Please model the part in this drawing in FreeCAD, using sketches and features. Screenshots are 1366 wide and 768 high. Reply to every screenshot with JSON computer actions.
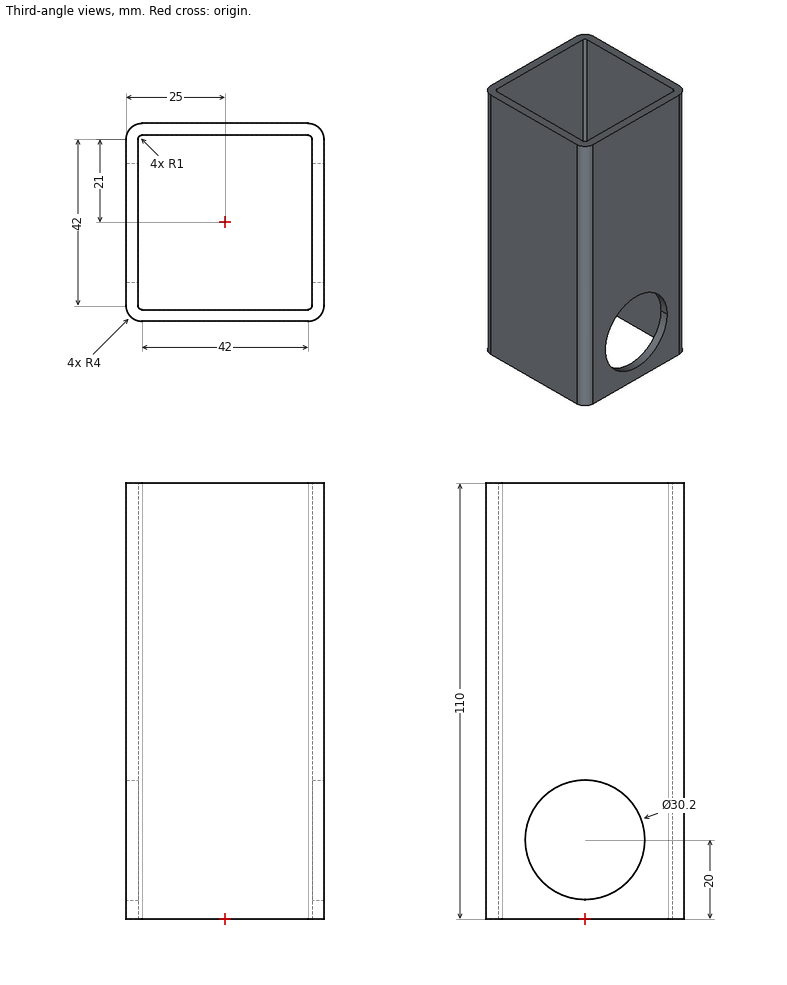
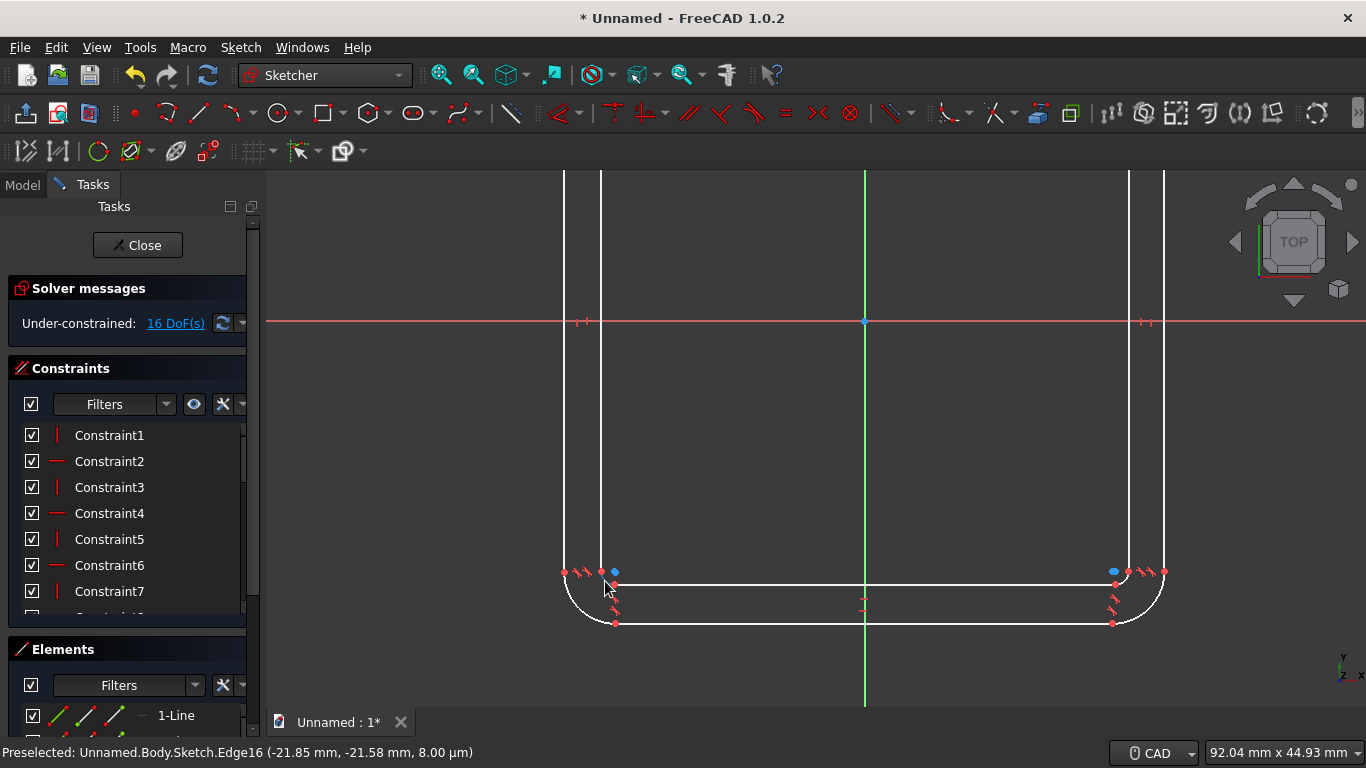
{"action": "left_click", "coordinate": [597, 279]}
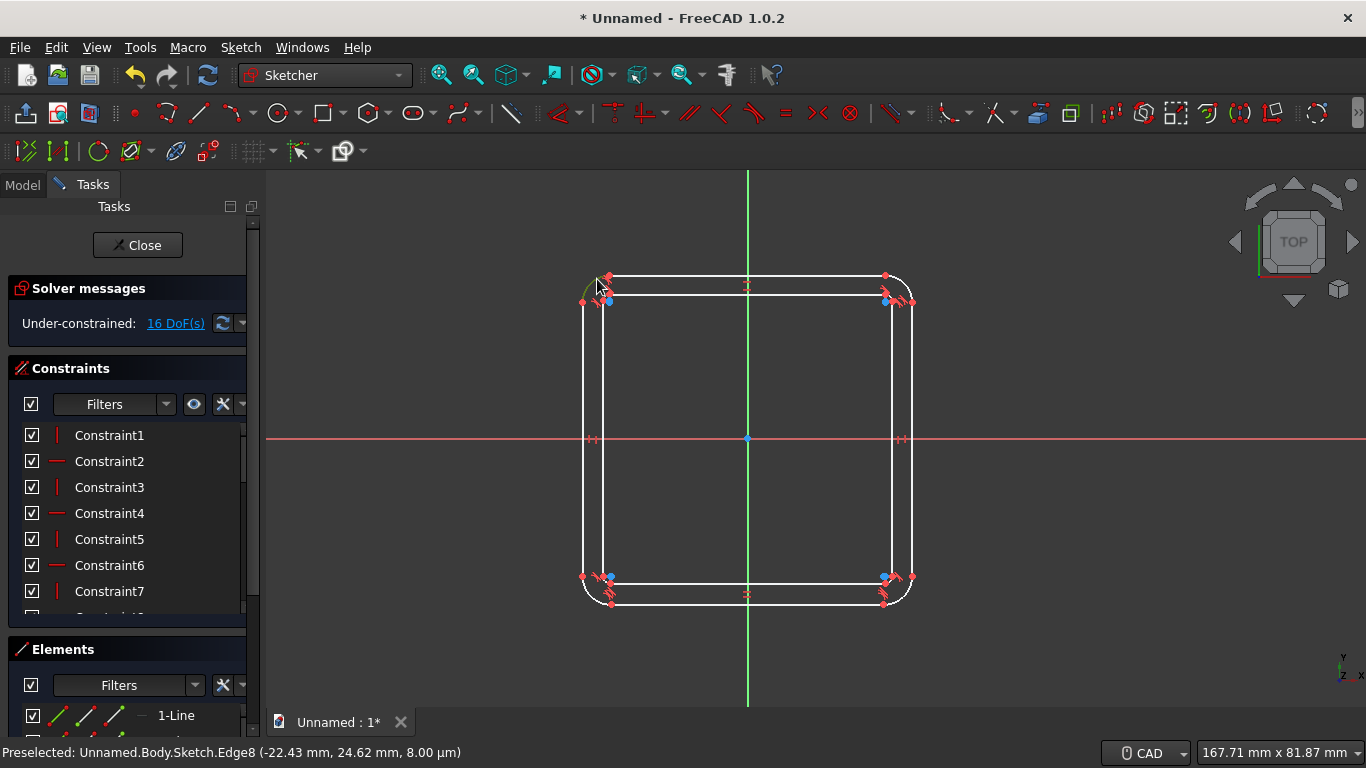
{"action": "scroll", "coordinate": [605, 296], "scroll_direction": "up", "scroll_amount": 6}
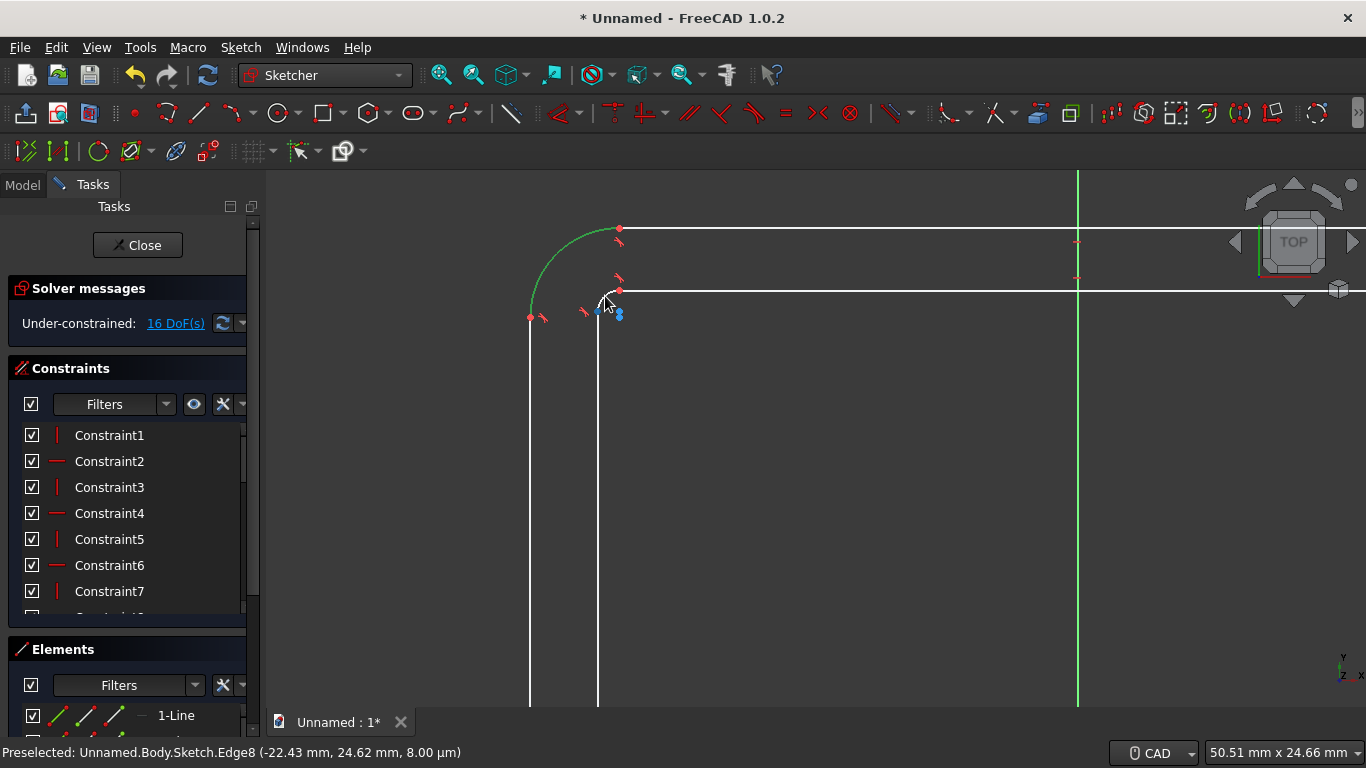
{"action": "left_click", "coordinate": [604, 297]}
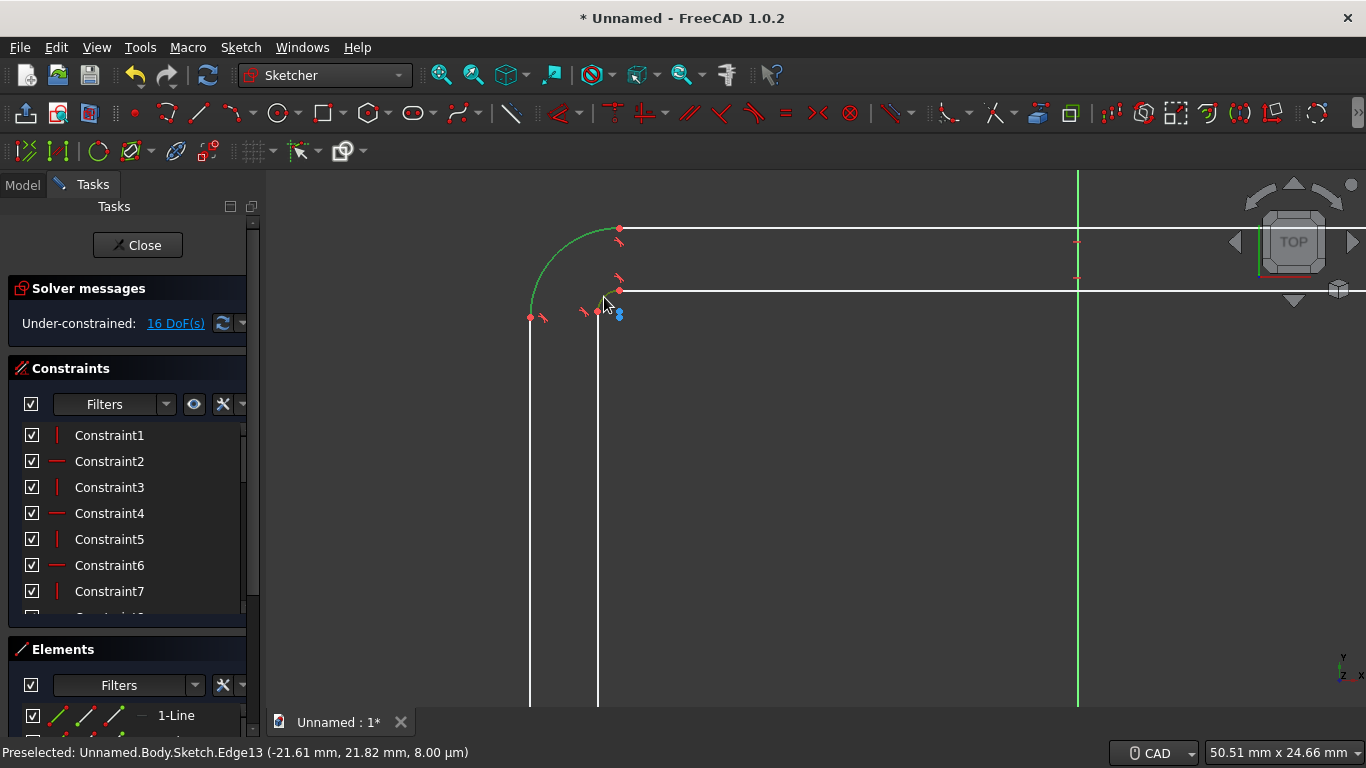
{"action": "left_click", "coordinate": [614, 114]}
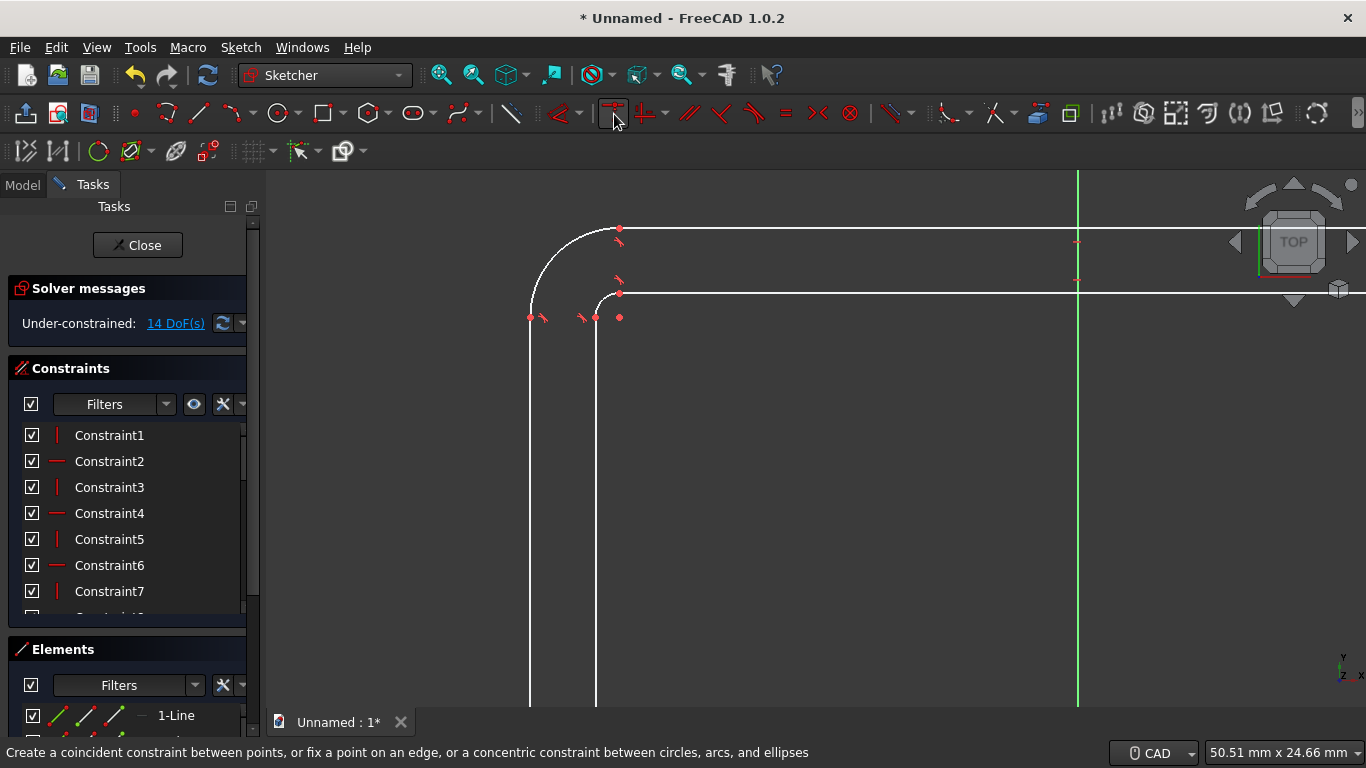
{"action": "scroll", "coordinate": [605, 296], "scroll_direction": "down", "scroll_amount": 6}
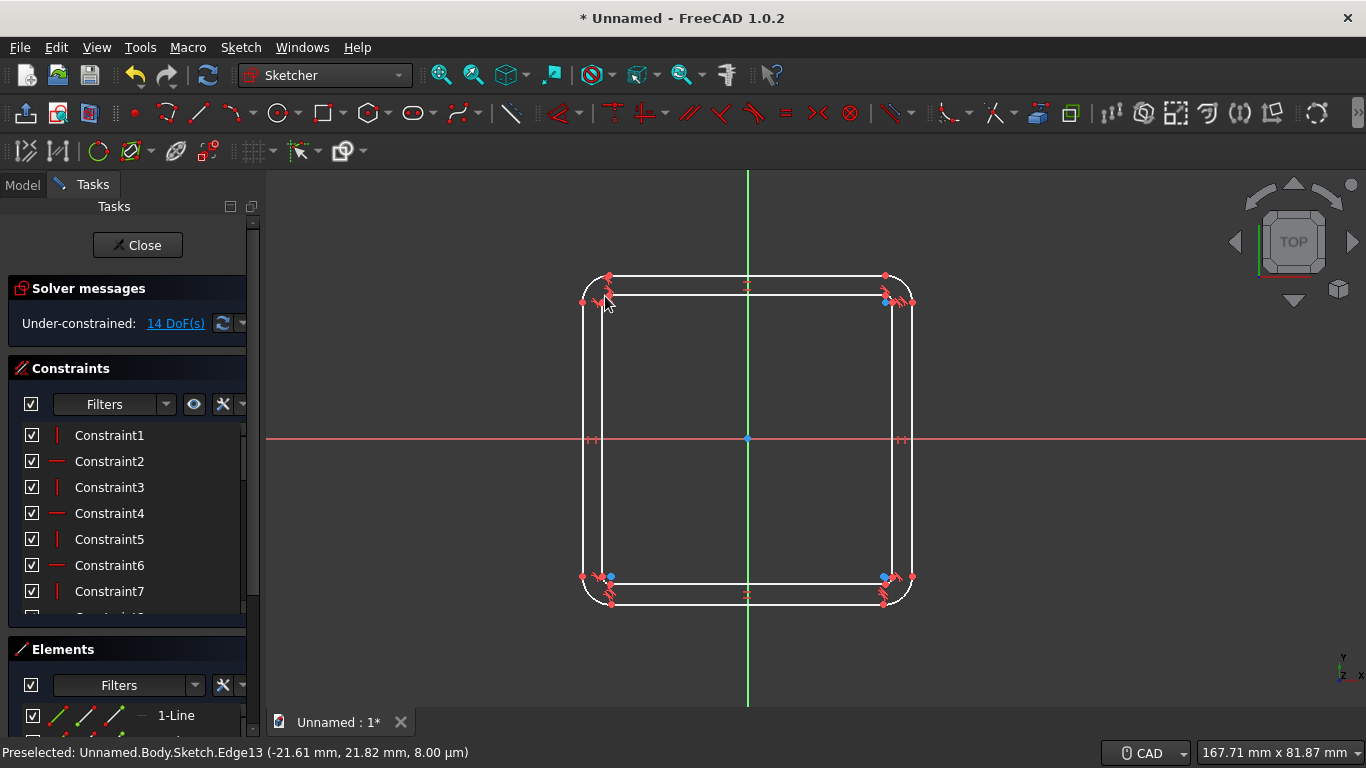
{"action": "left_click", "coordinate": [909, 290]}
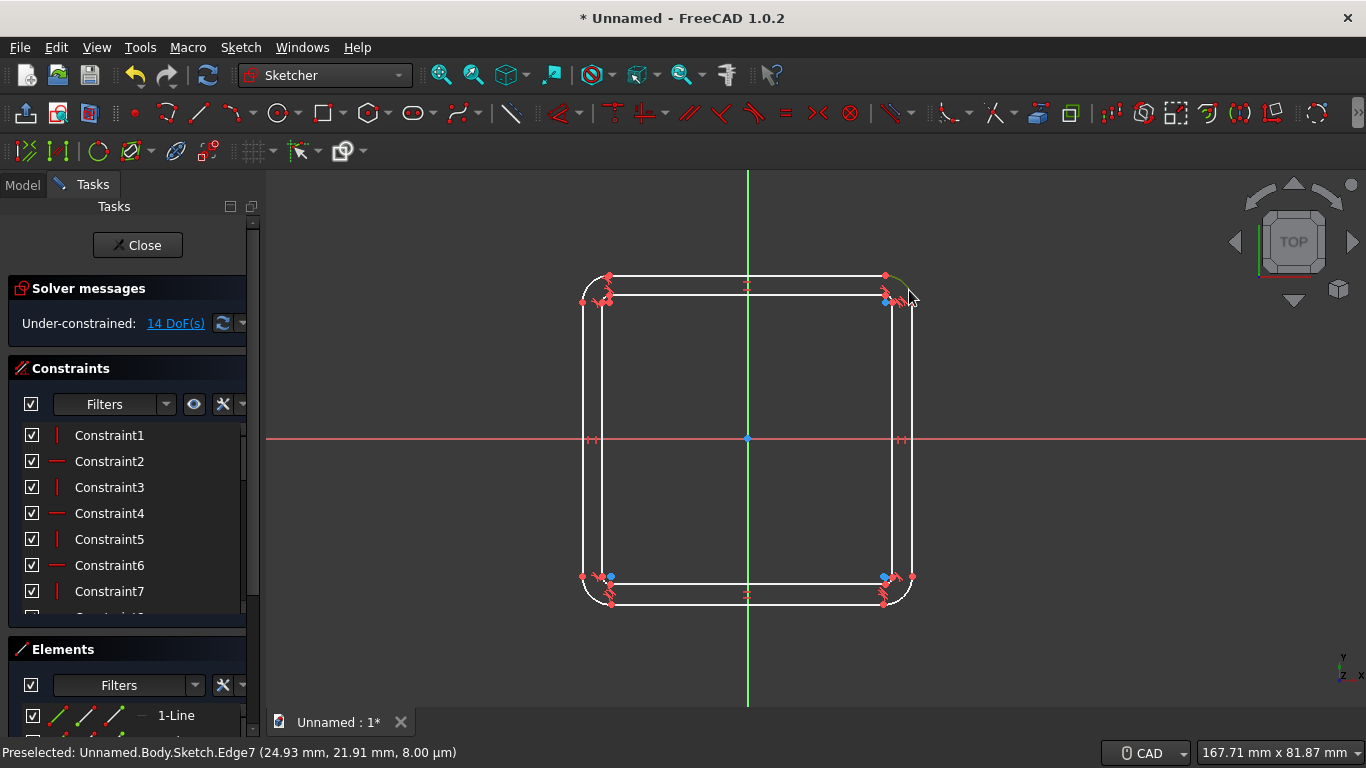
{"action": "scroll", "coordinate": [890, 297], "scroll_direction": "up", "scroll_amount": 5}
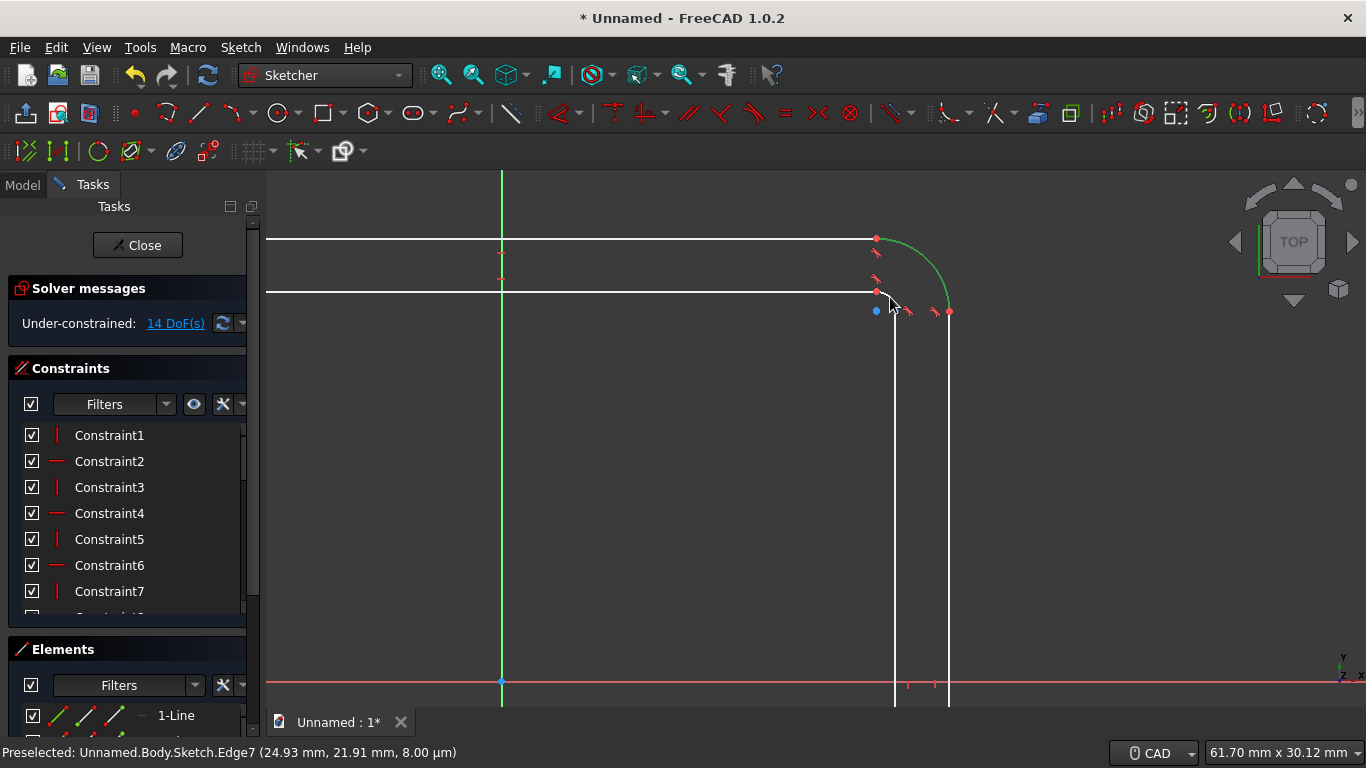
{"action": "left_click", "coordinate": [890, 297]}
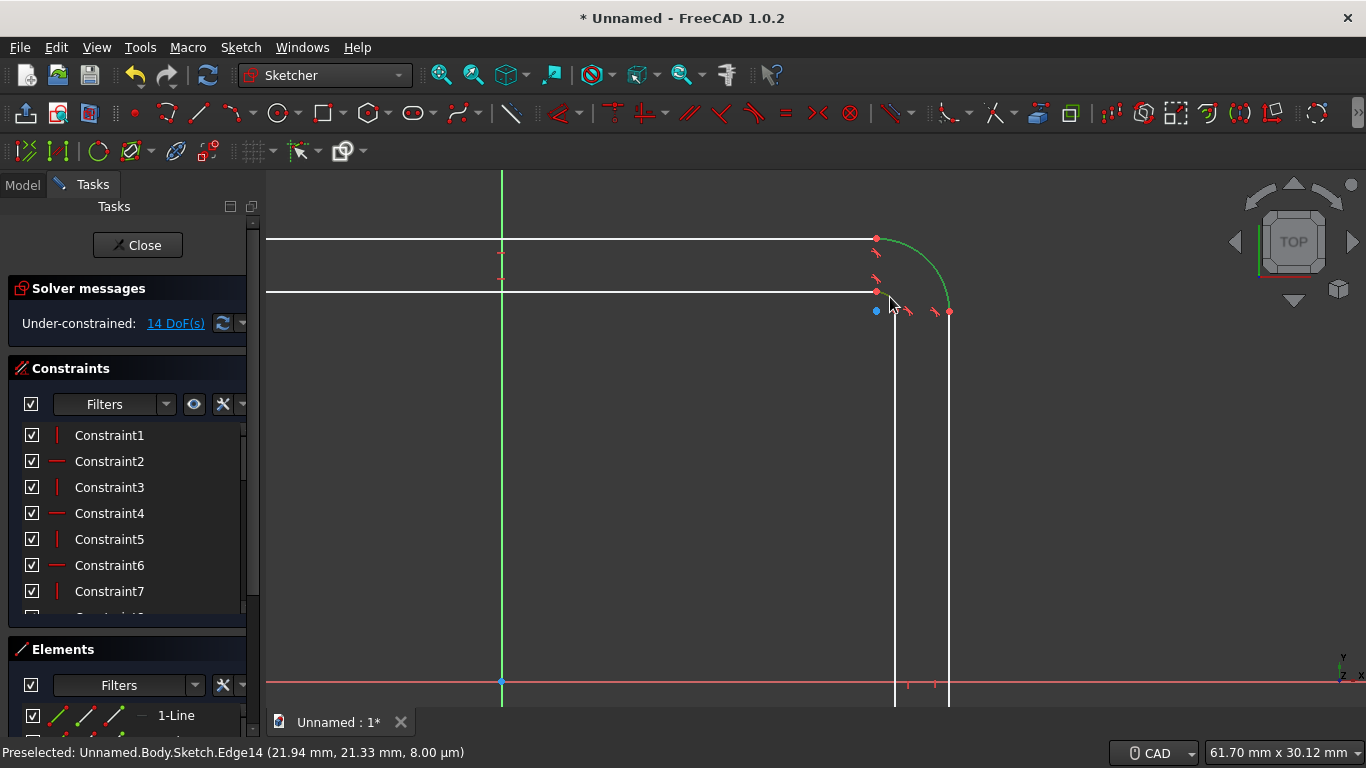
{"action": "left_click", "coordinate": [614, 114]}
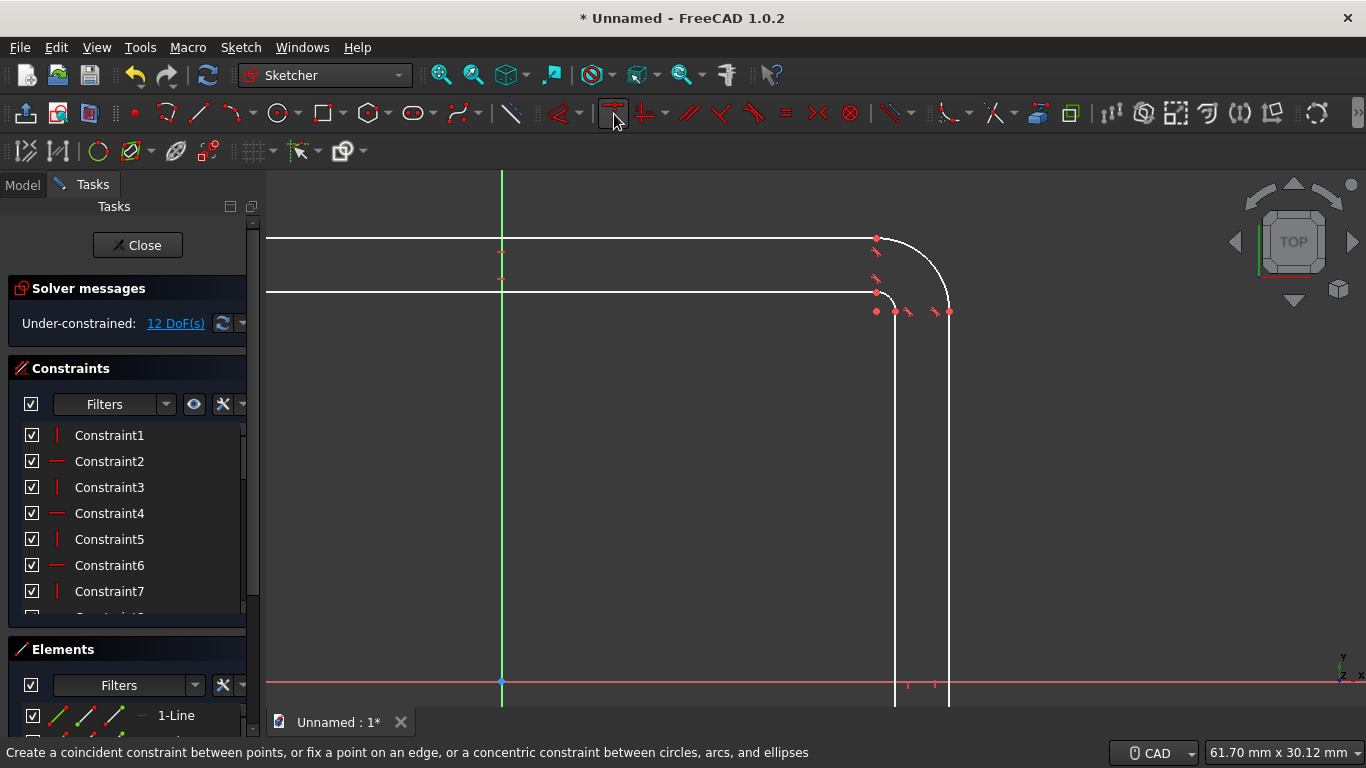
{"action": "scroll", "coordinate": [890, 297], "scroll_direction": "down", "scroll_amount": 5}